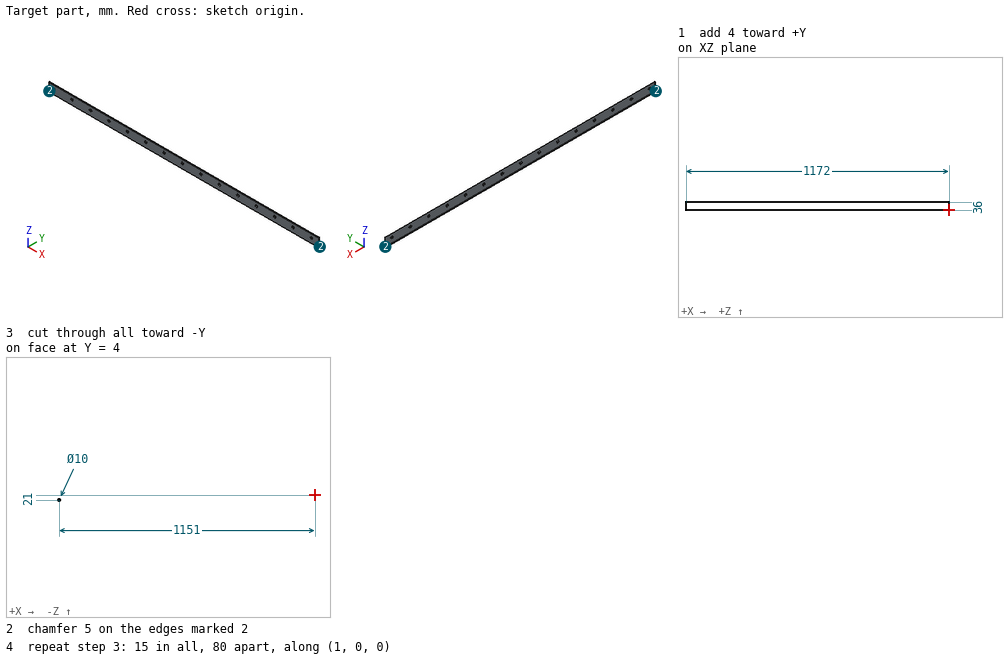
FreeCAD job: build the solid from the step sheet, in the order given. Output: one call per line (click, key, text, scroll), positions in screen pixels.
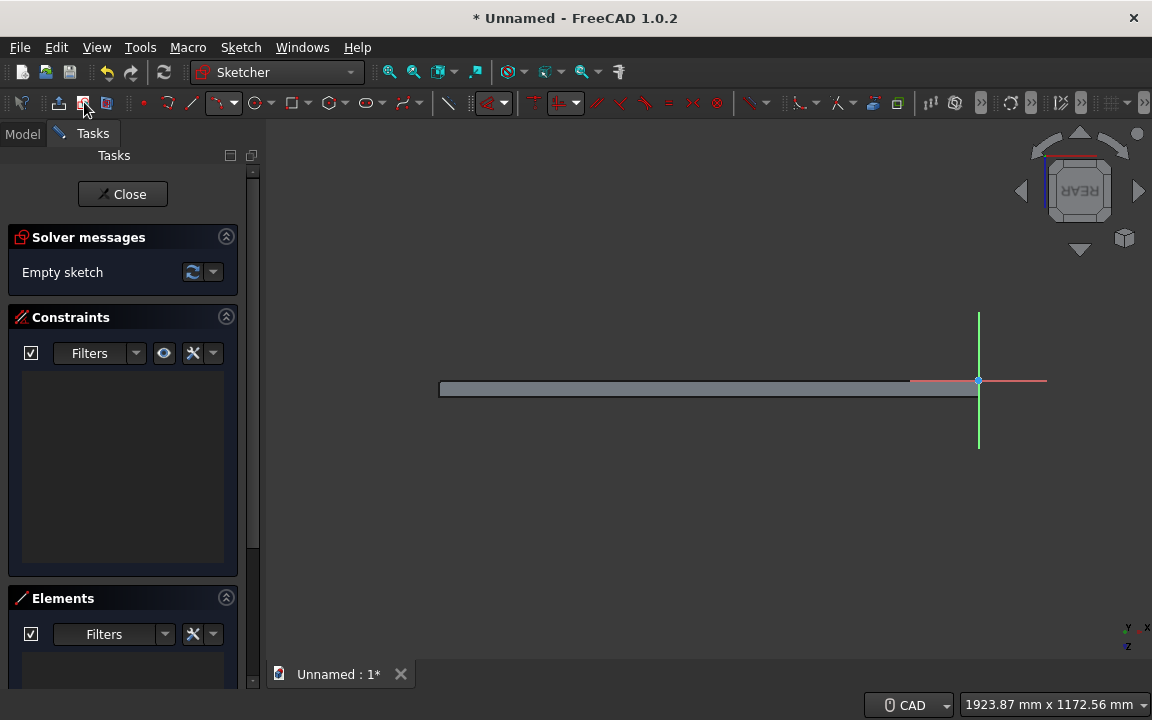
scroll(439, 390, up, 15)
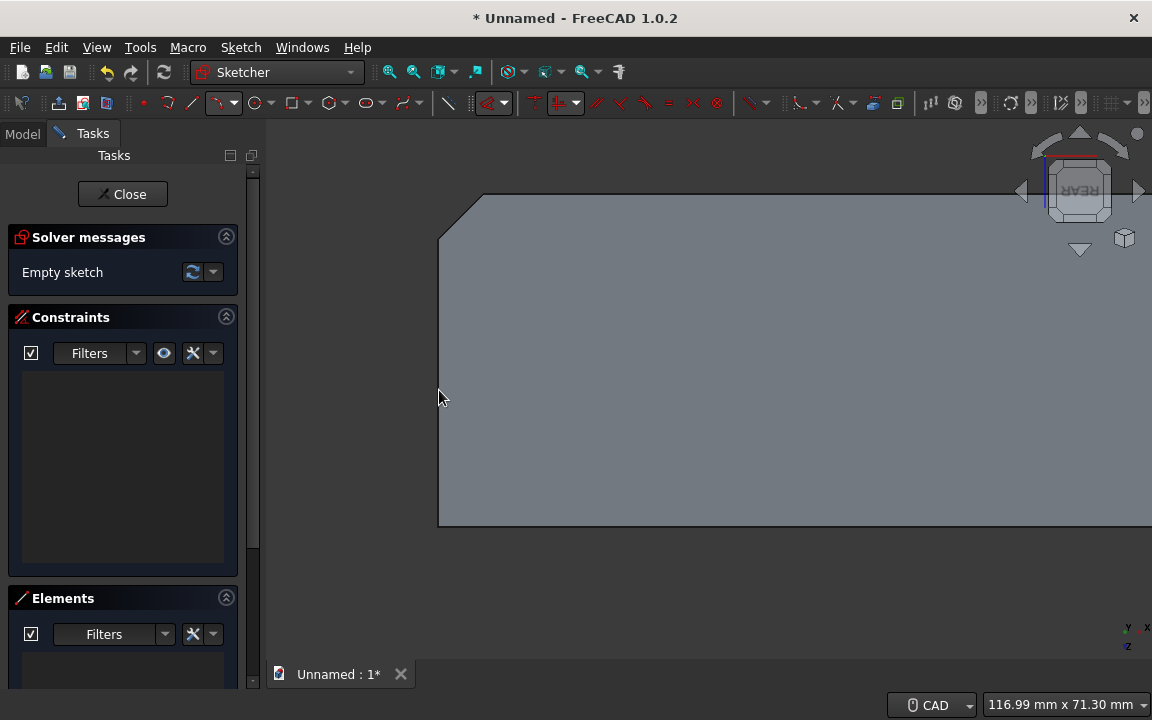
scroll(629, 388, up, 7)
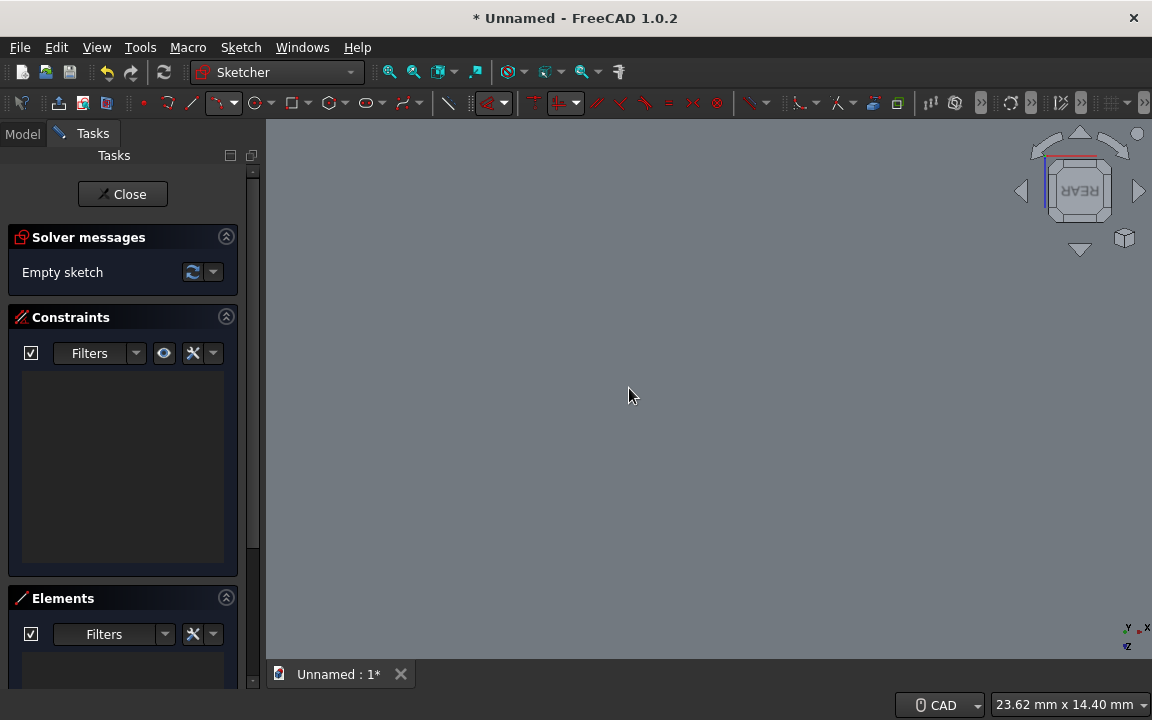
click(256, 104)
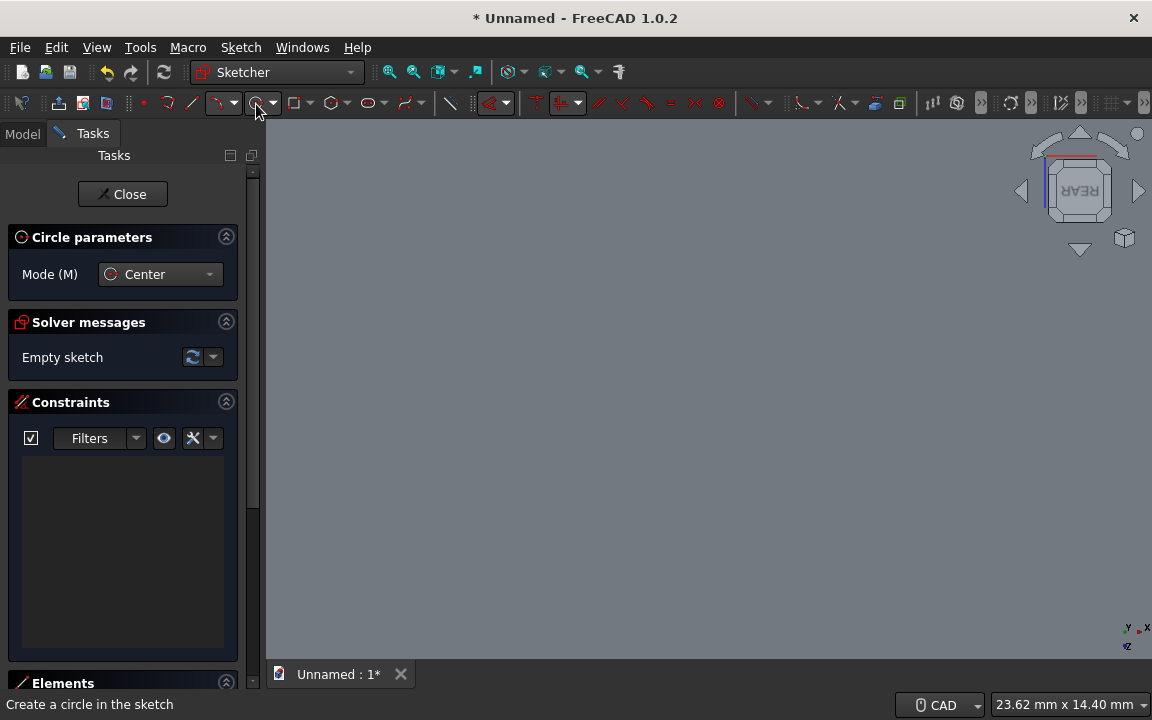
click(640, 387)
click(773, 254)
key(Escape)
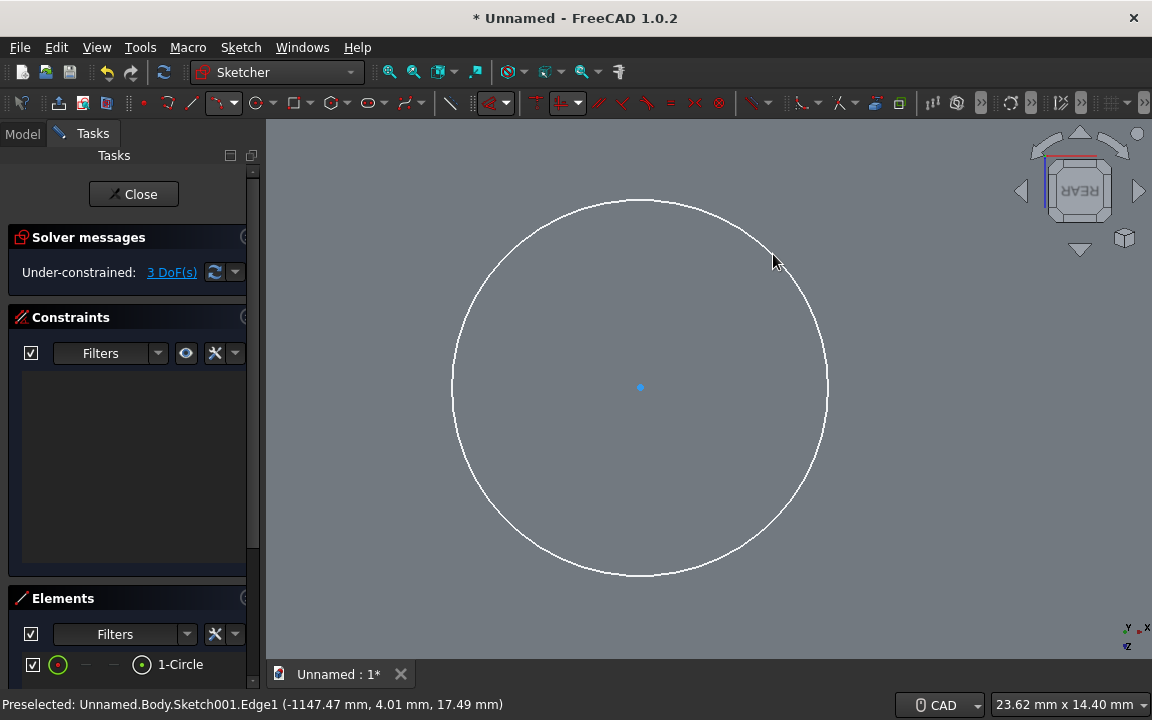
click(773, 255)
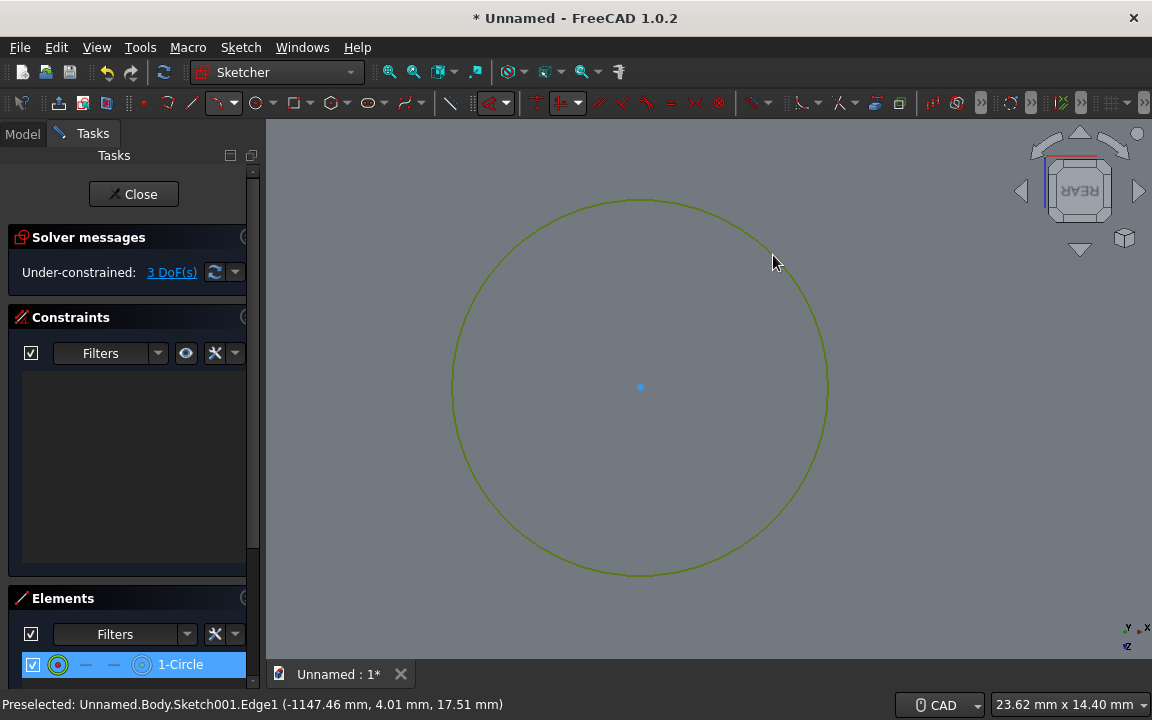
key(k)
key(o)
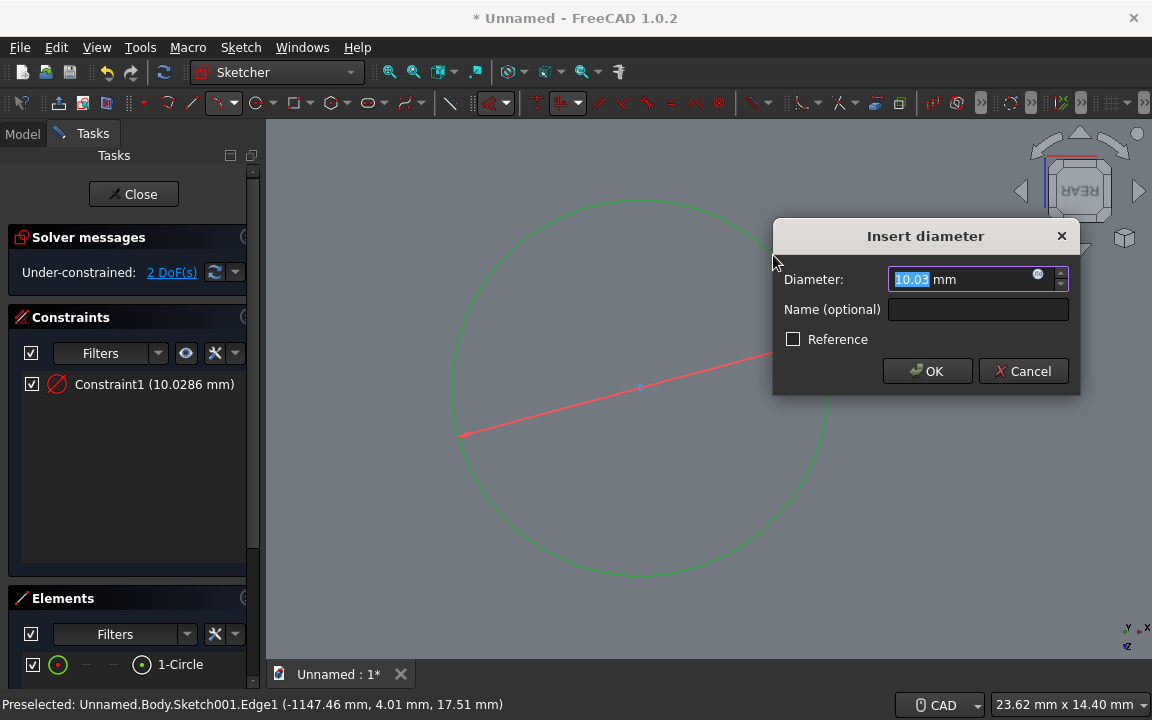
text(10)
key(Return)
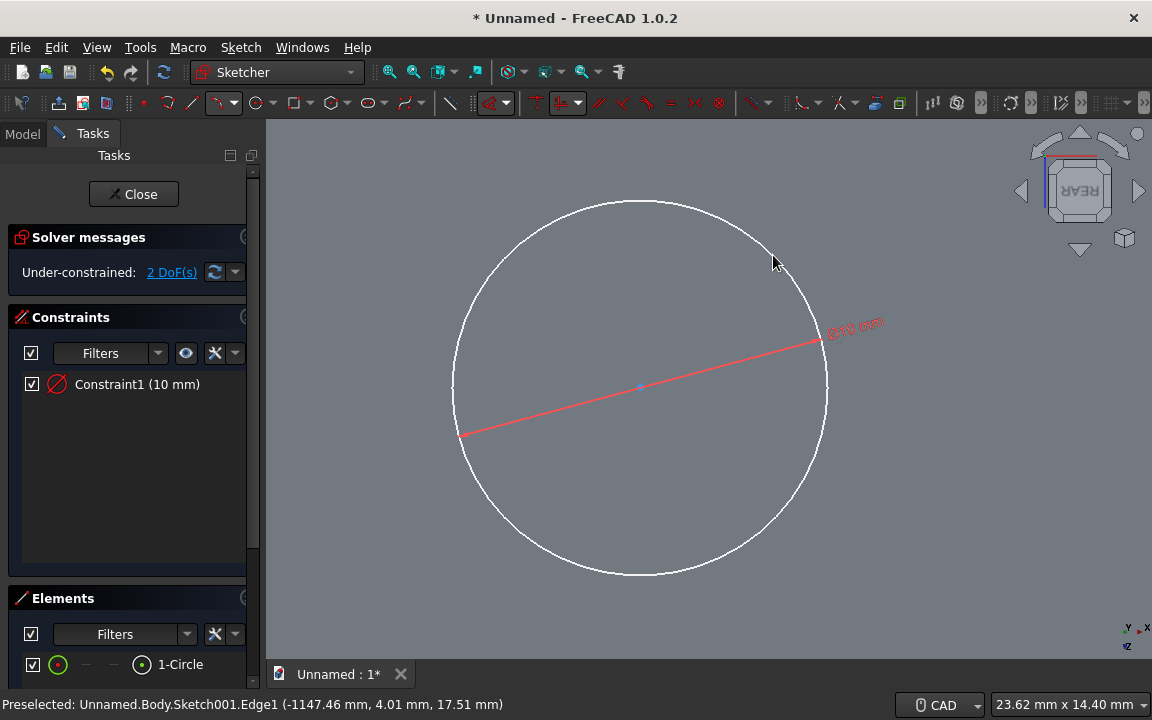
click(640, 388)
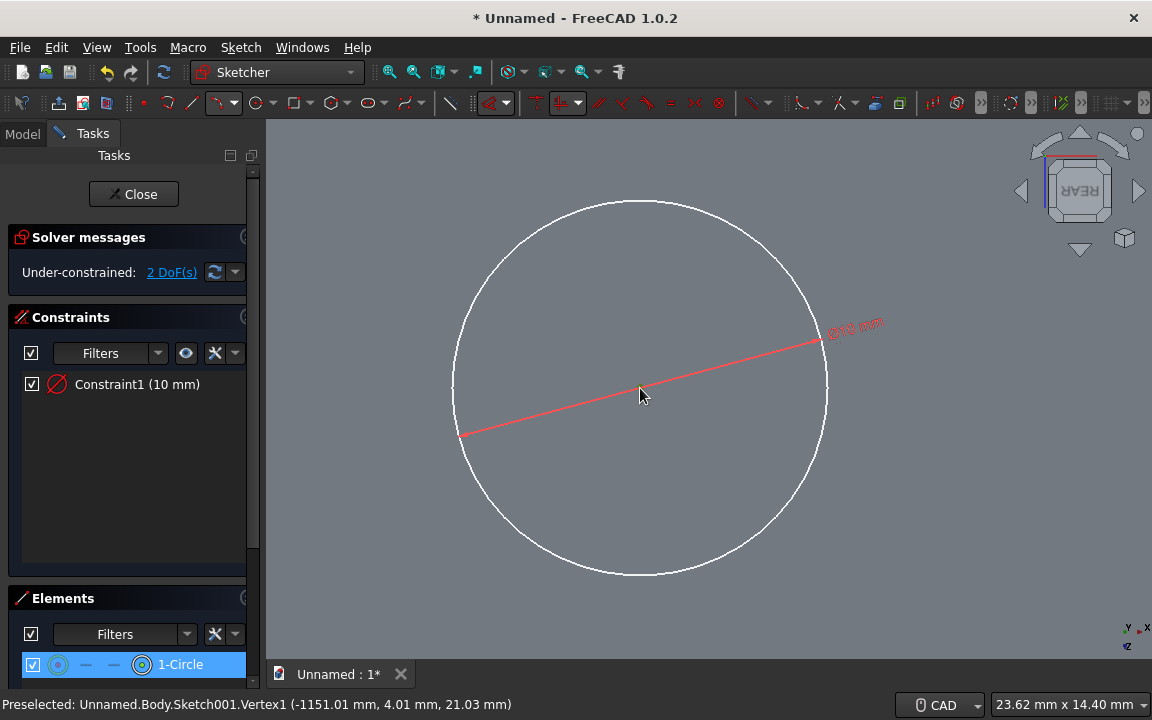
click(508, 104)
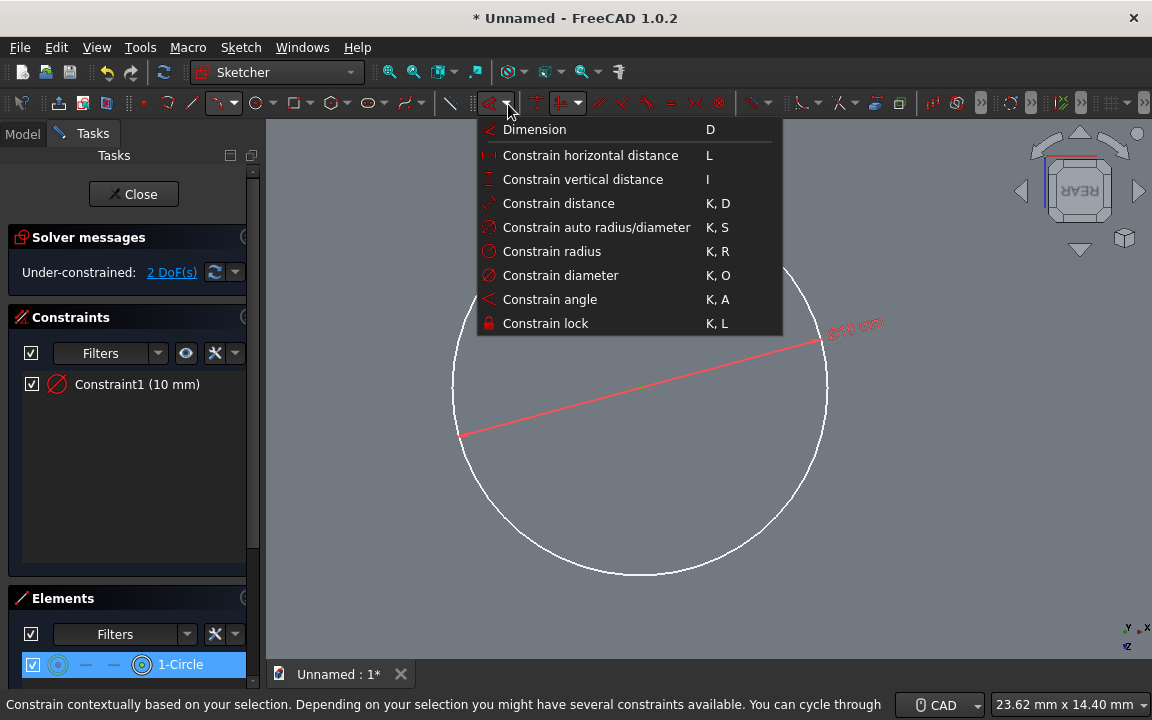
click(630, 179)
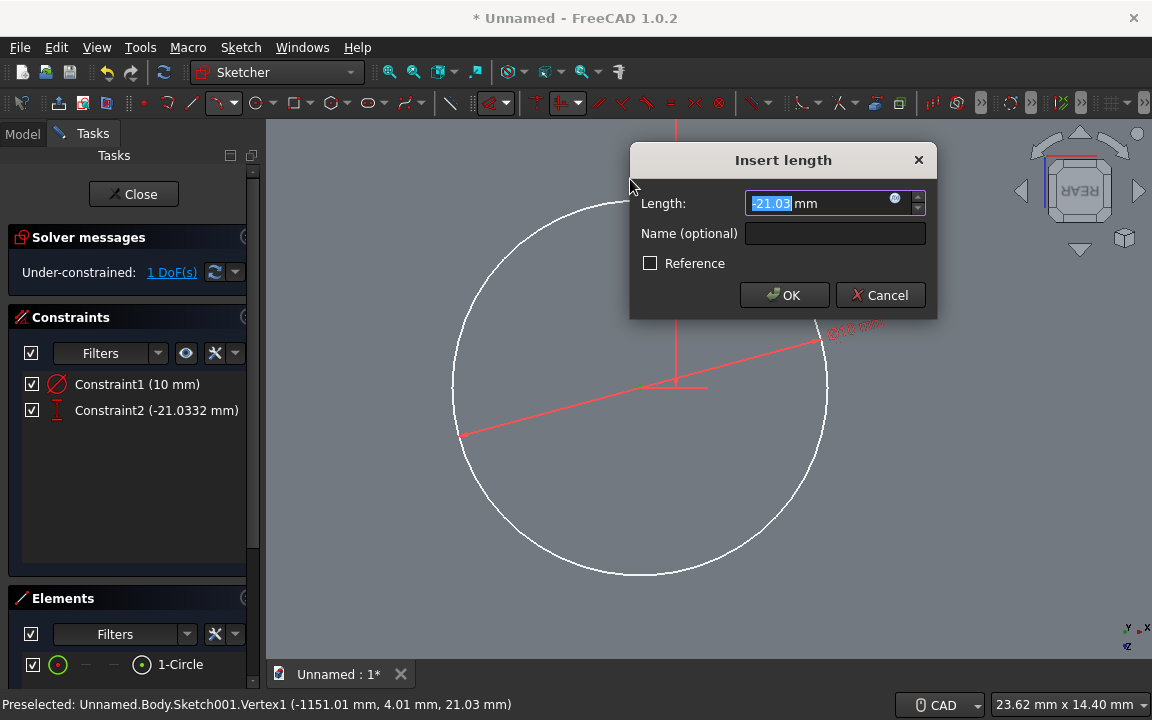
text(-21)
key(Return)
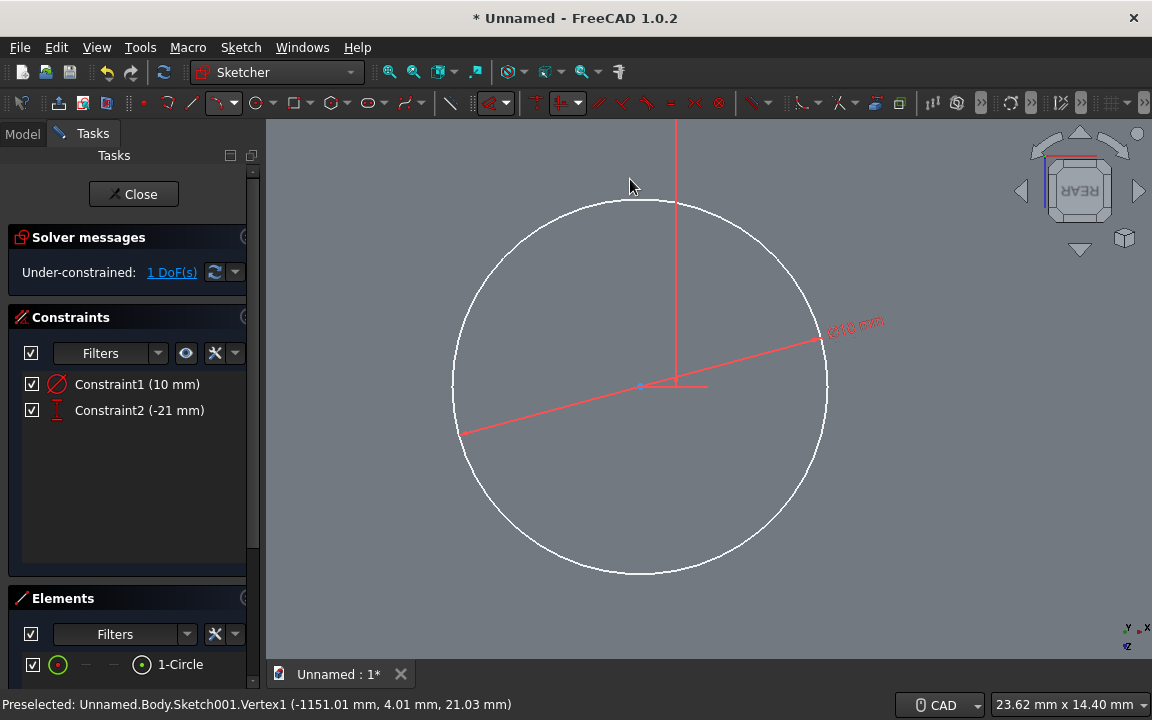
click(640, 387)